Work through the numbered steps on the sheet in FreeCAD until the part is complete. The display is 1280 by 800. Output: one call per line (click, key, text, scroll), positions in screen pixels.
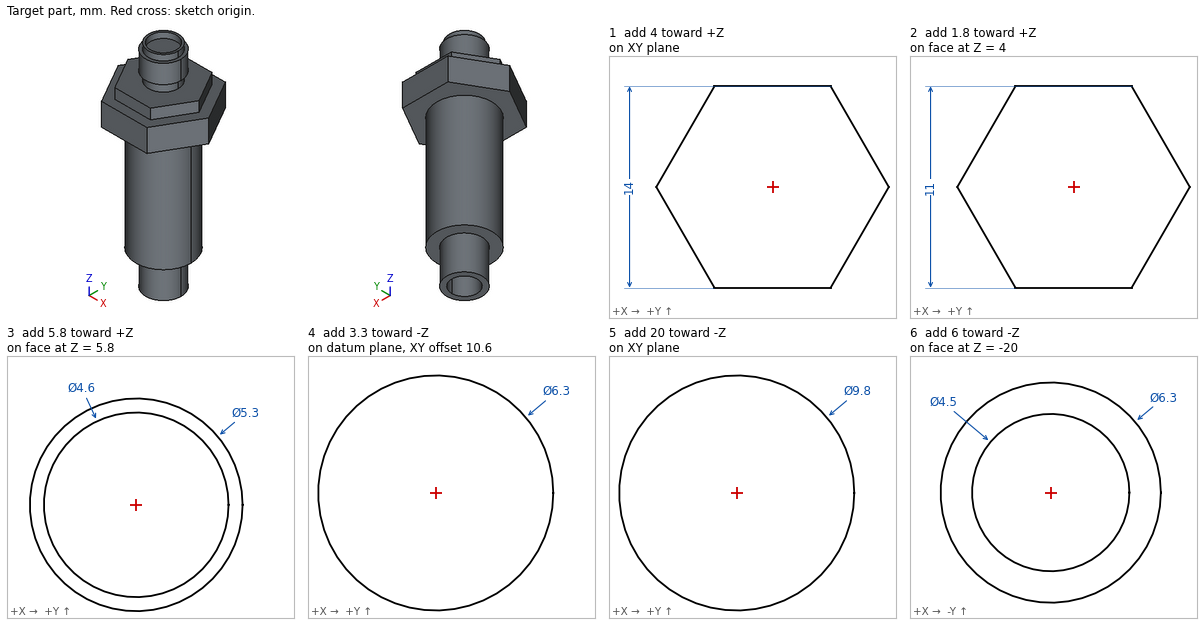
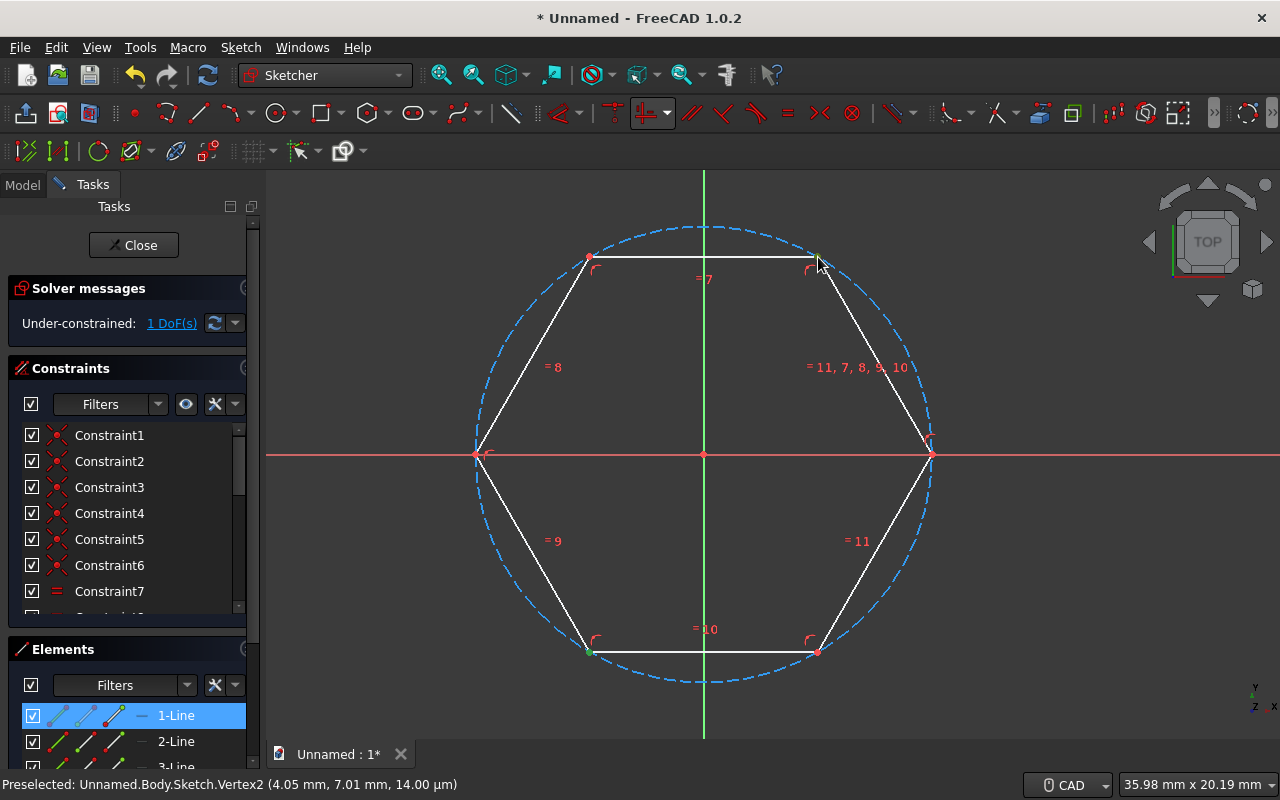
click(582, 114)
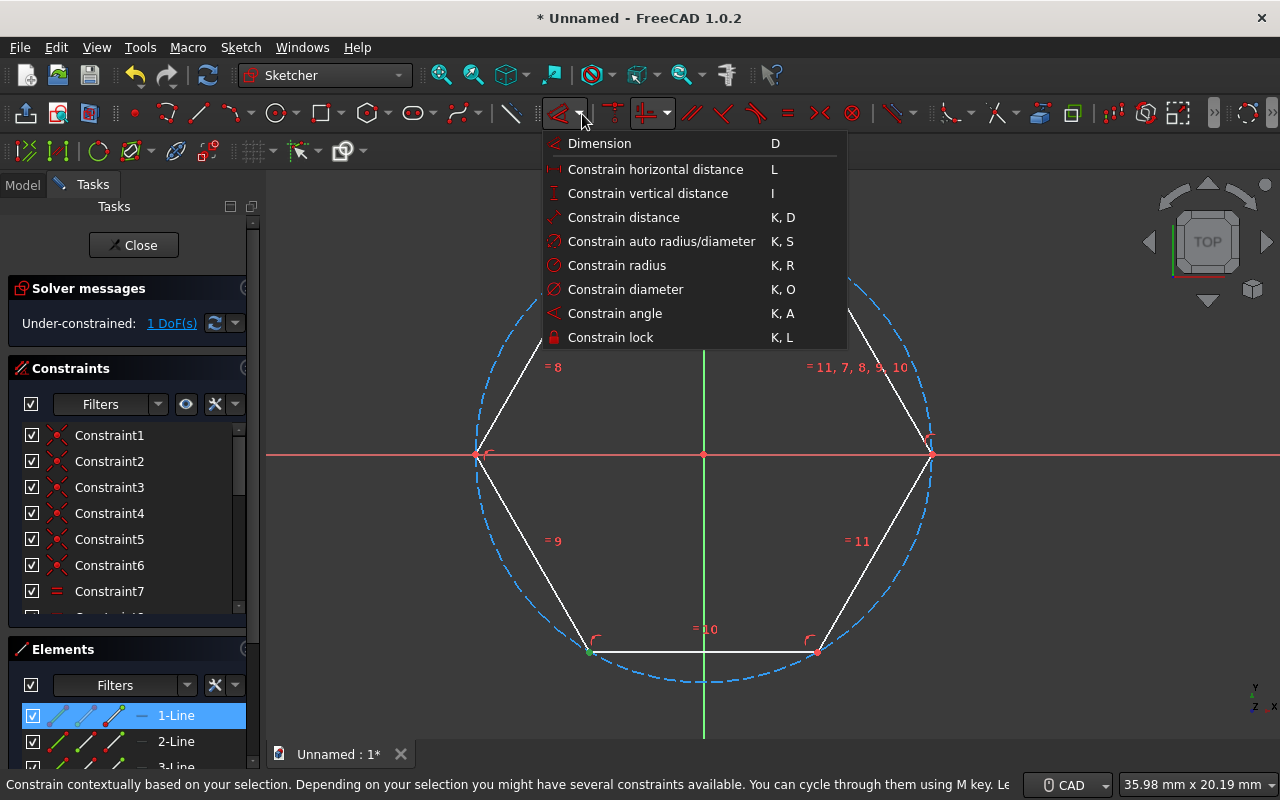
click(695, 193)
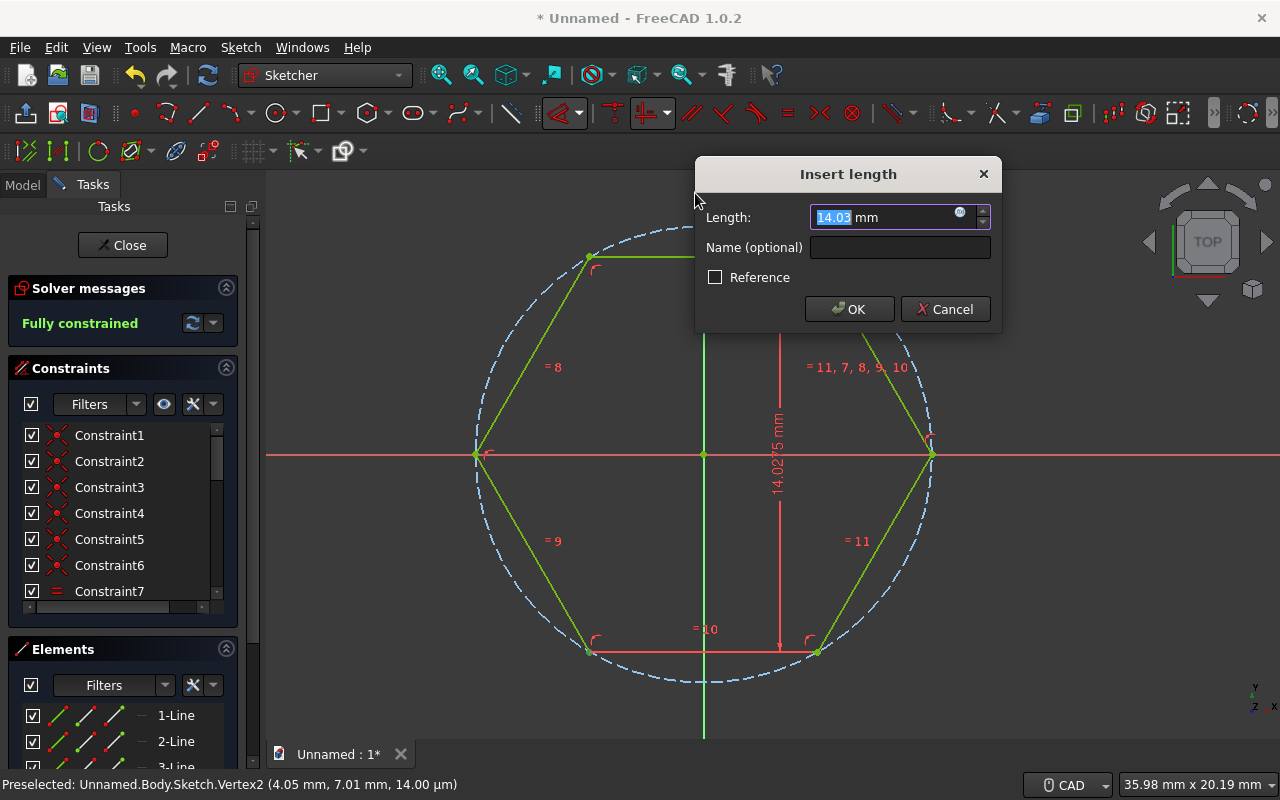
text(14)
key(Return)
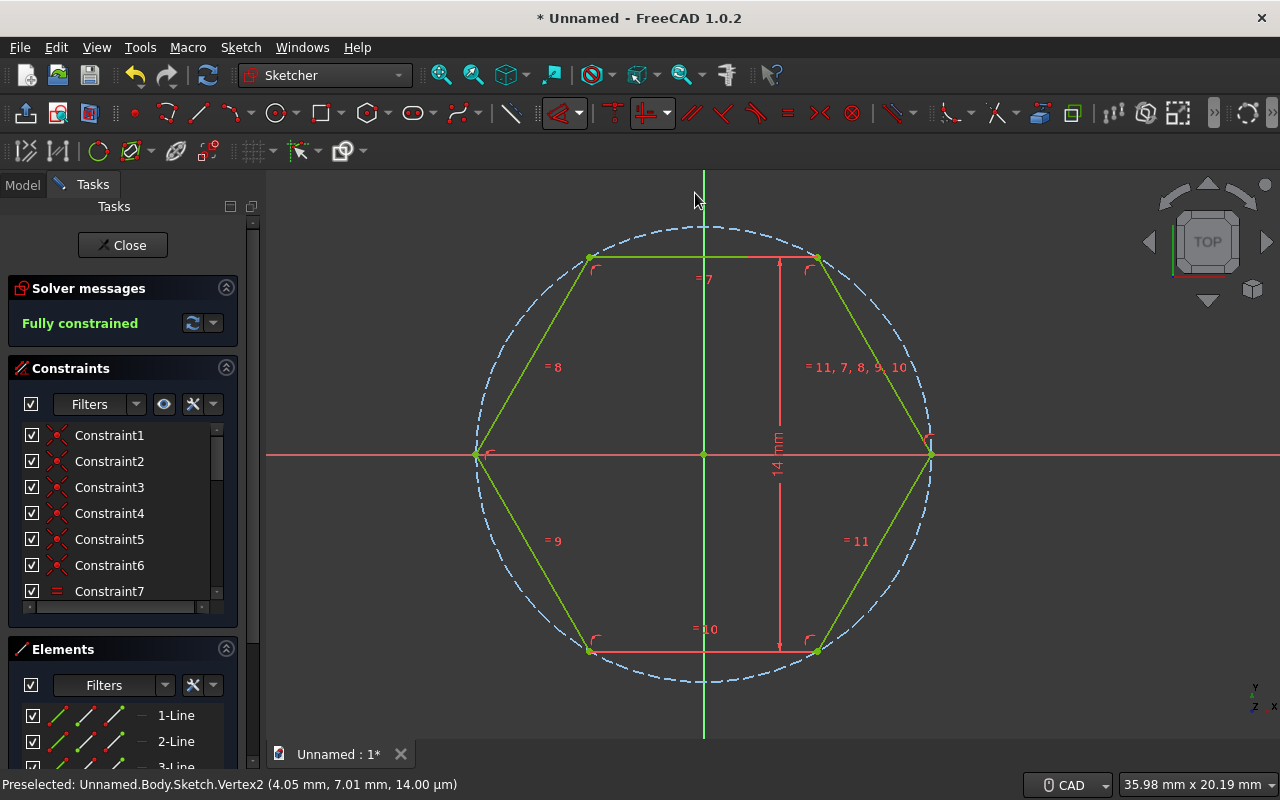
click(123, 245)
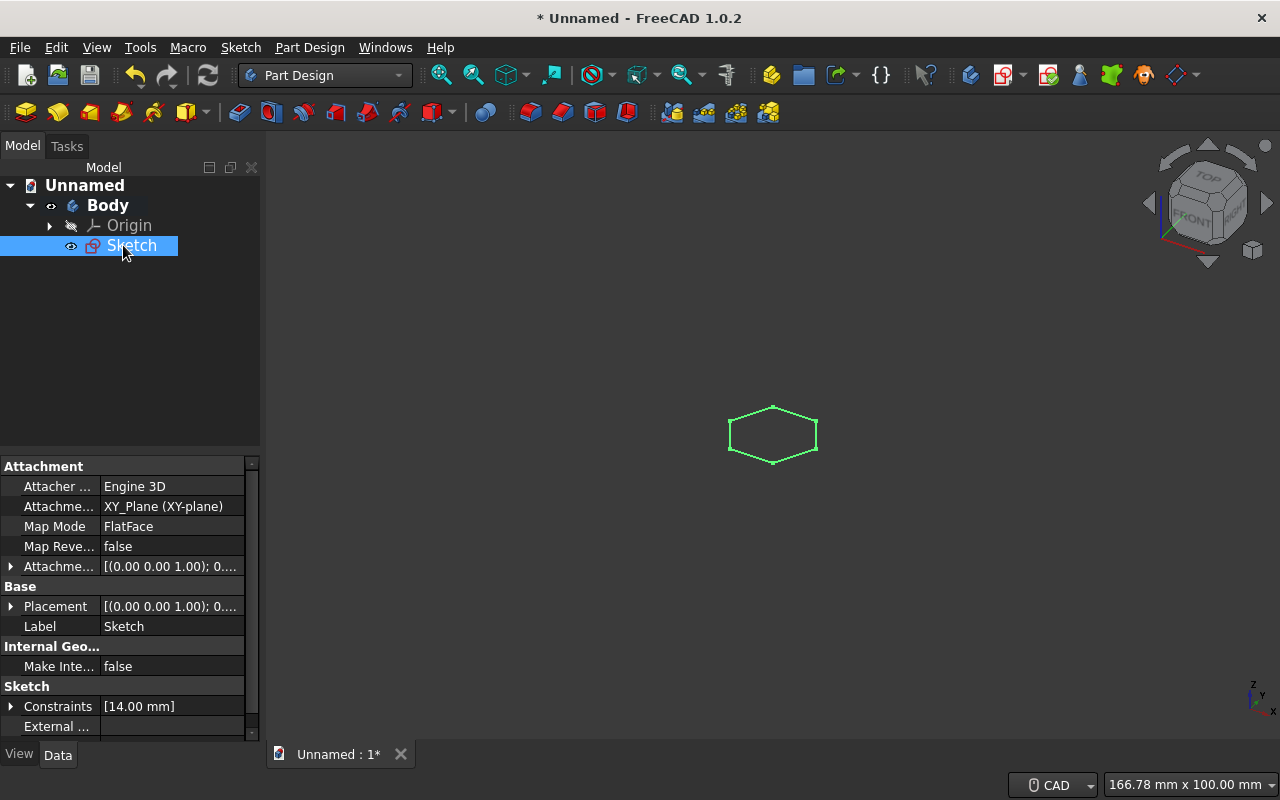
click(26, 112)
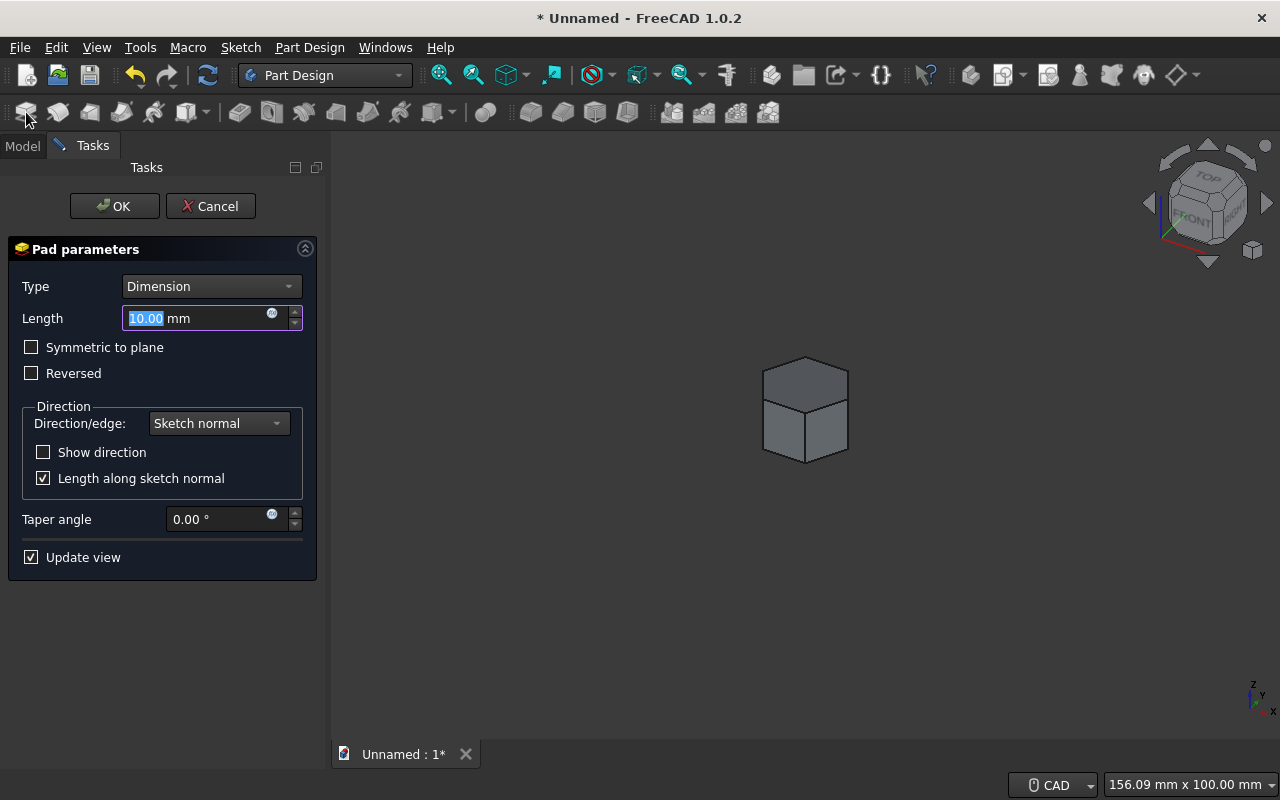
text(4)
key(Tab)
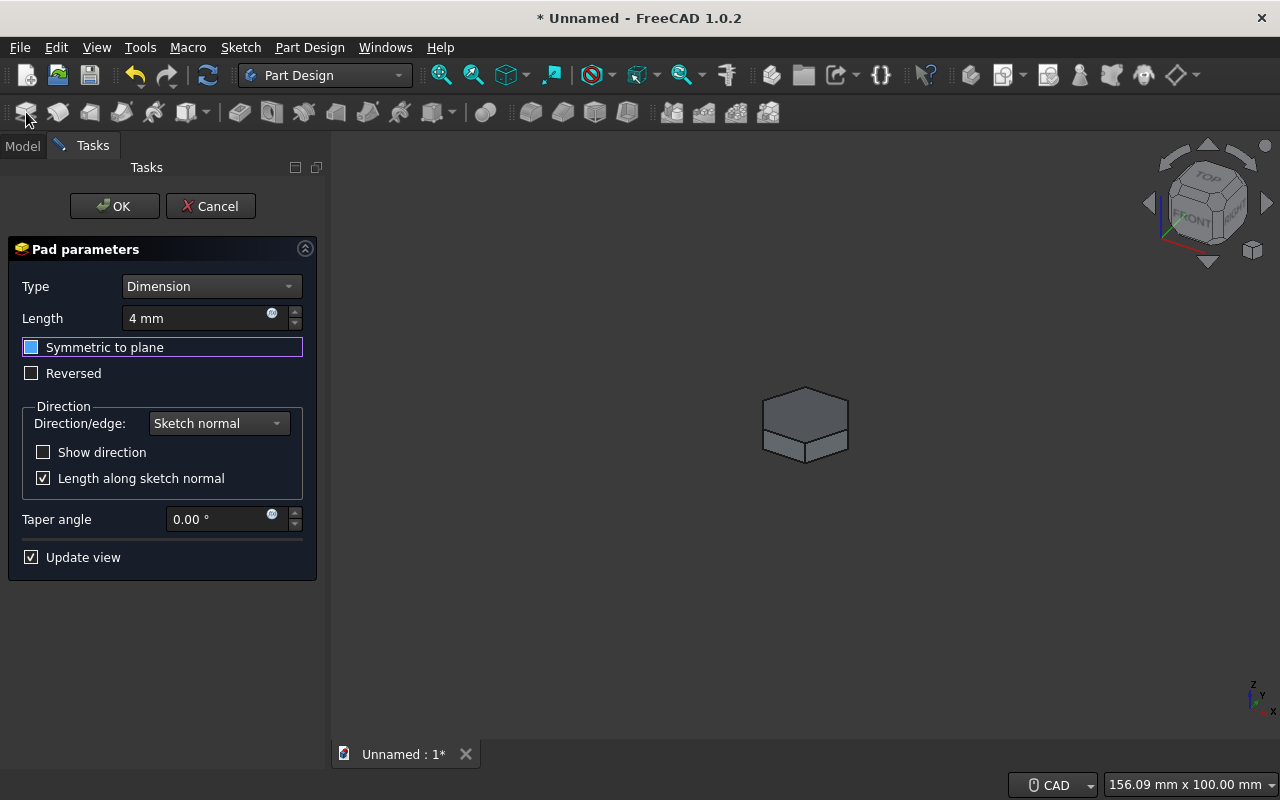
click(115, 206)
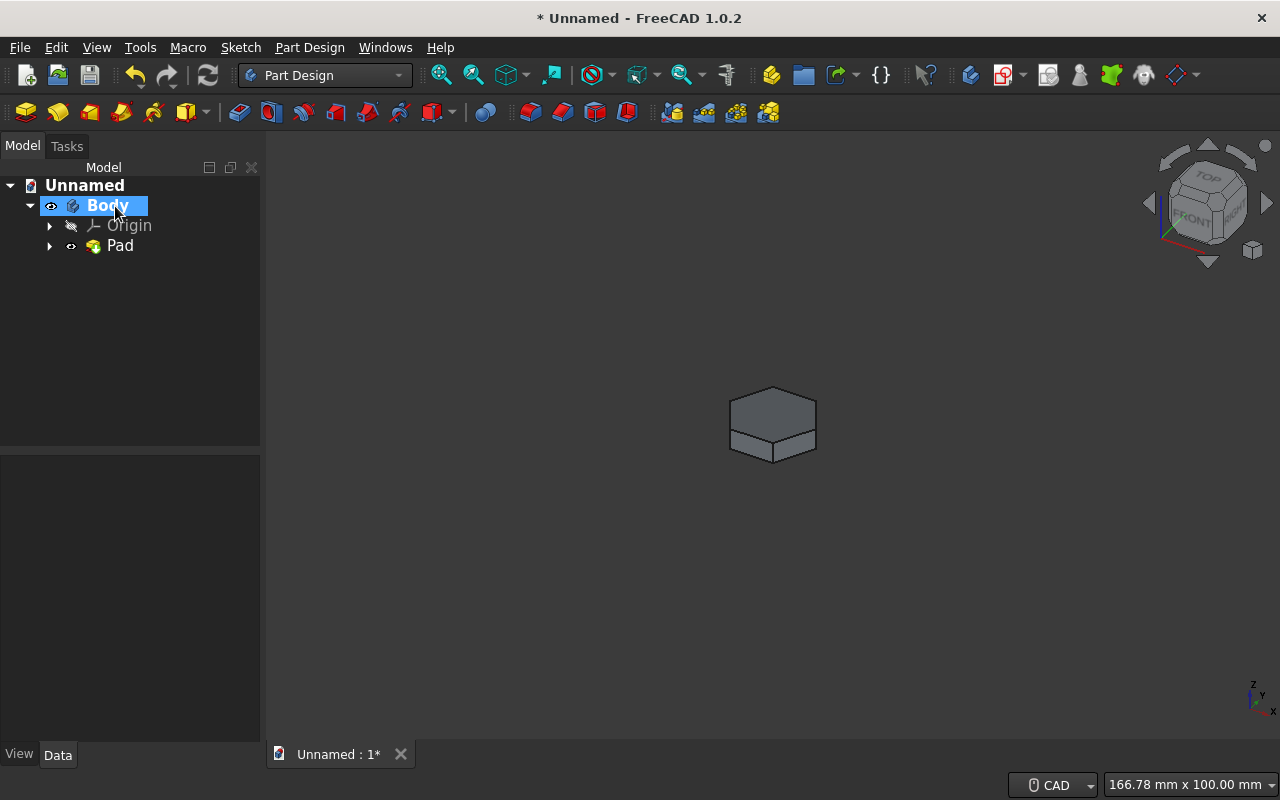
click(442, 76)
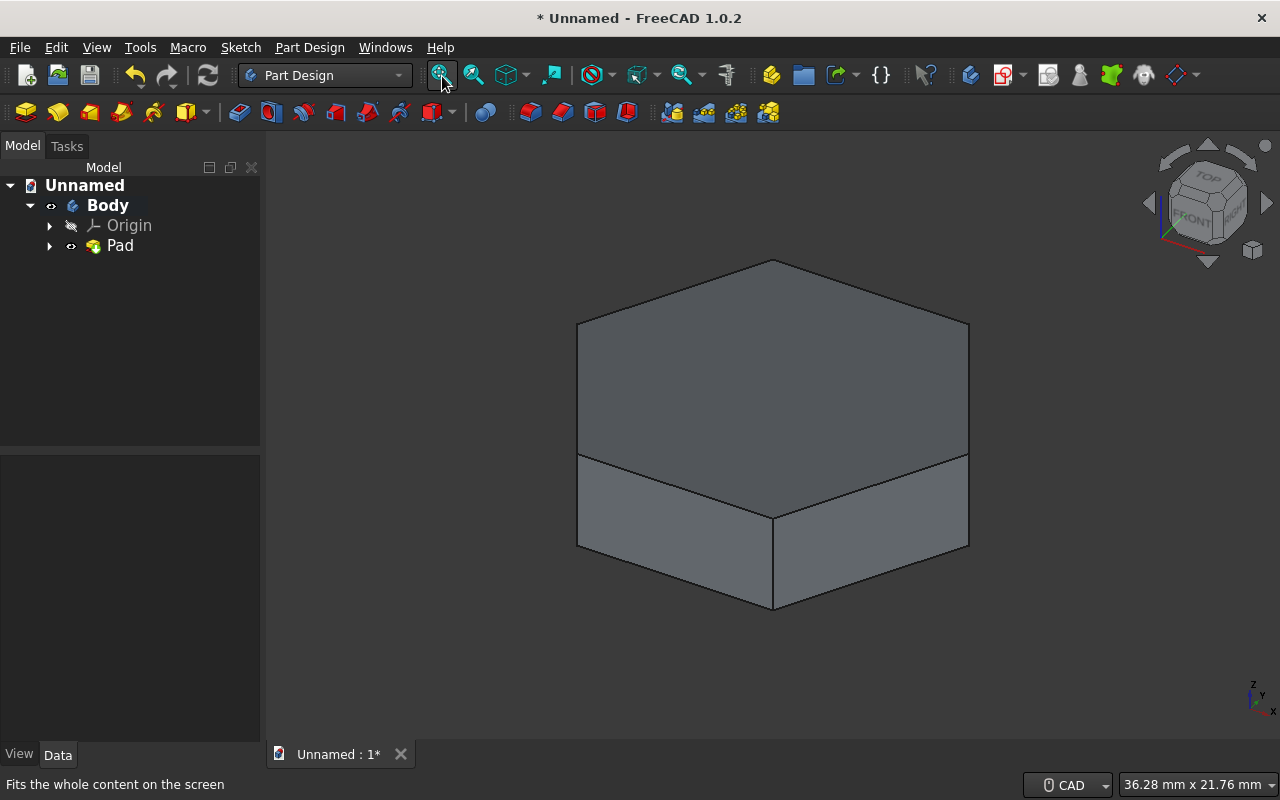
click(773, 388)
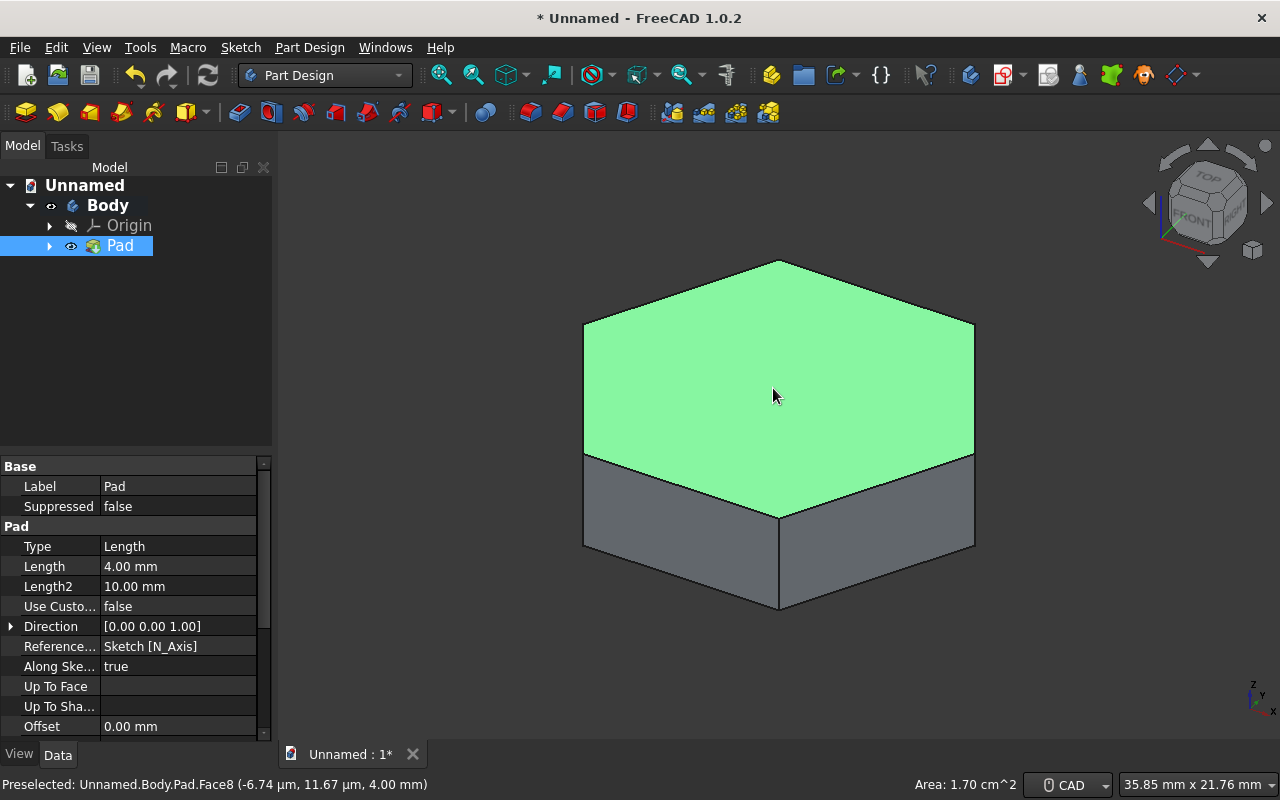
click(1004, 76)